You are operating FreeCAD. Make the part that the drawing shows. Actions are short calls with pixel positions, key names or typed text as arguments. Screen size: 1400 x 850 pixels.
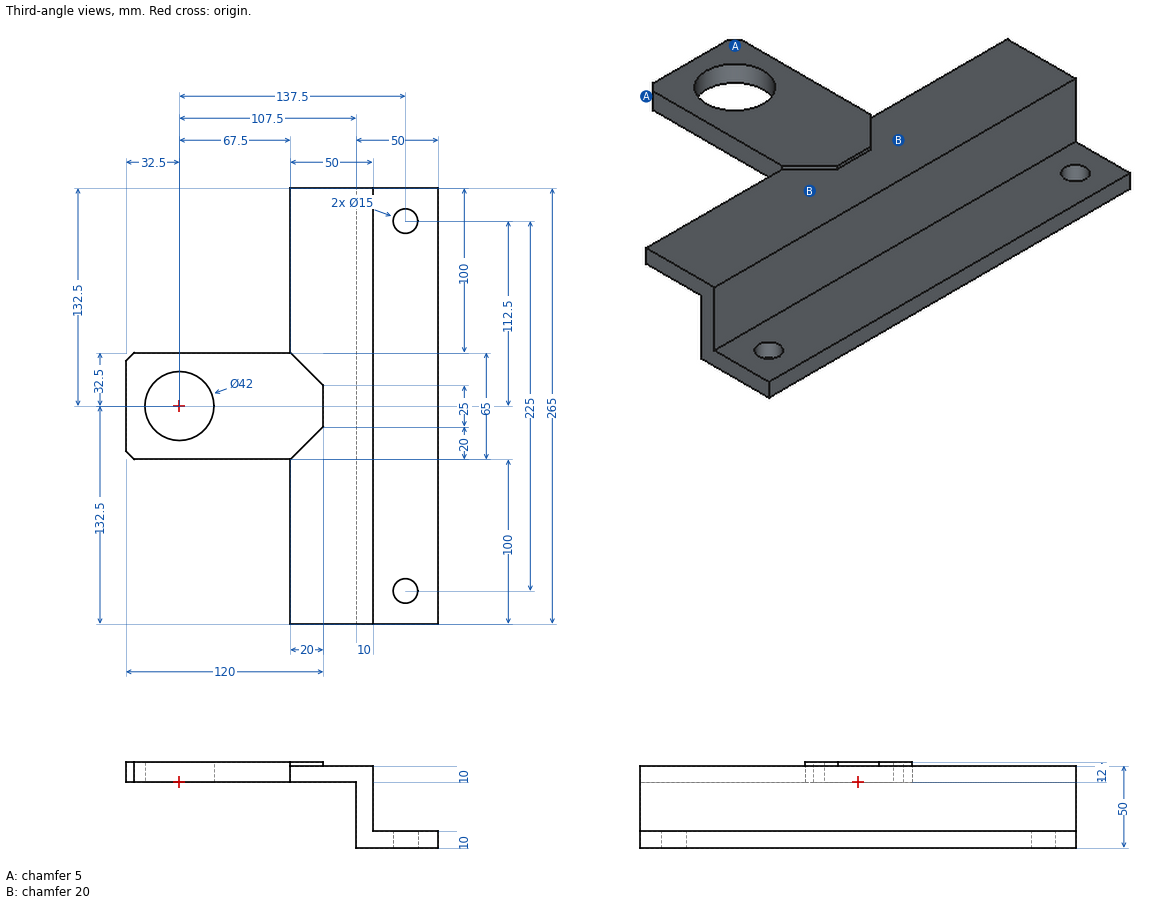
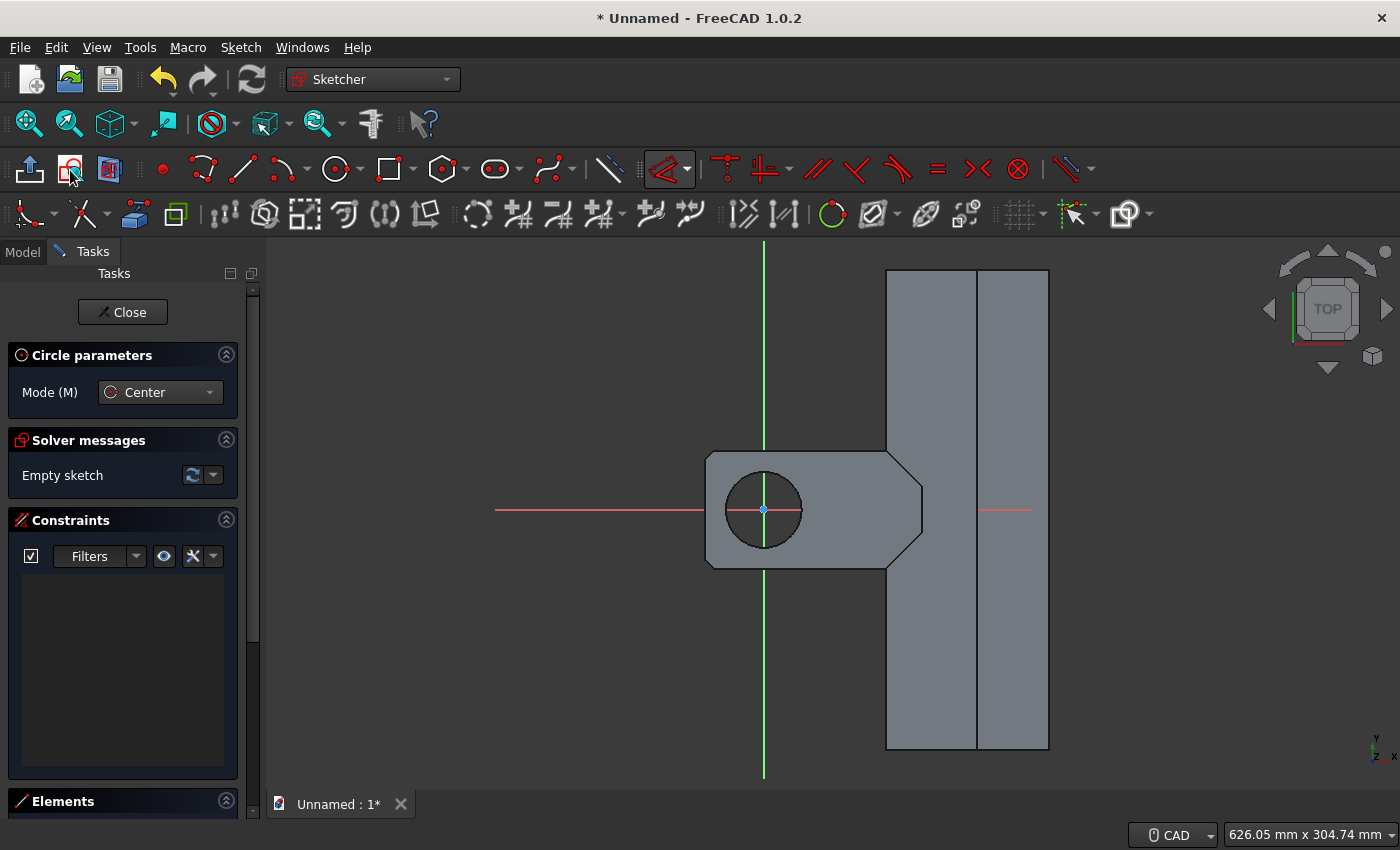
scroll(1013, 306, up, 3)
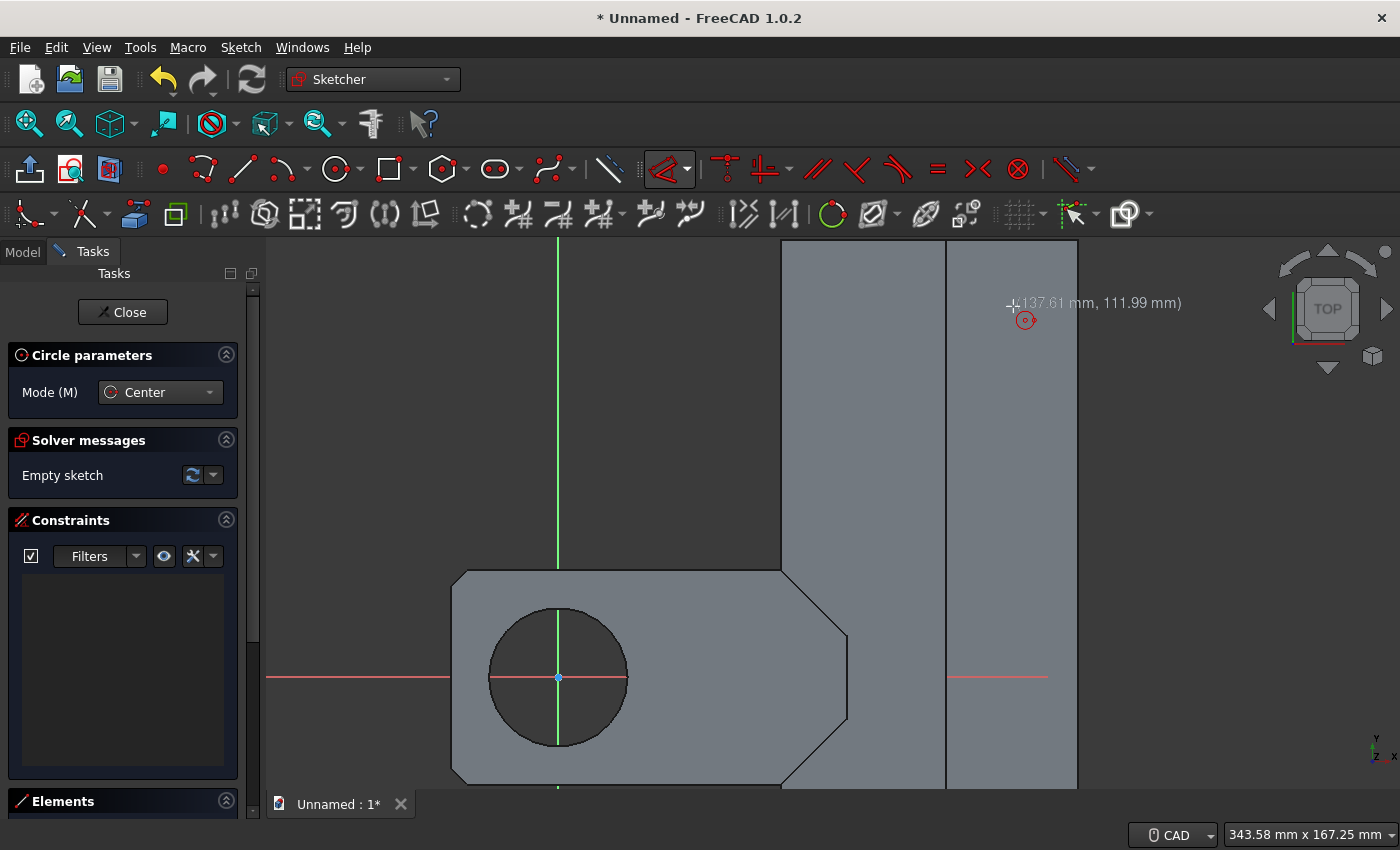
click(1012, 306)
move(1030, 289)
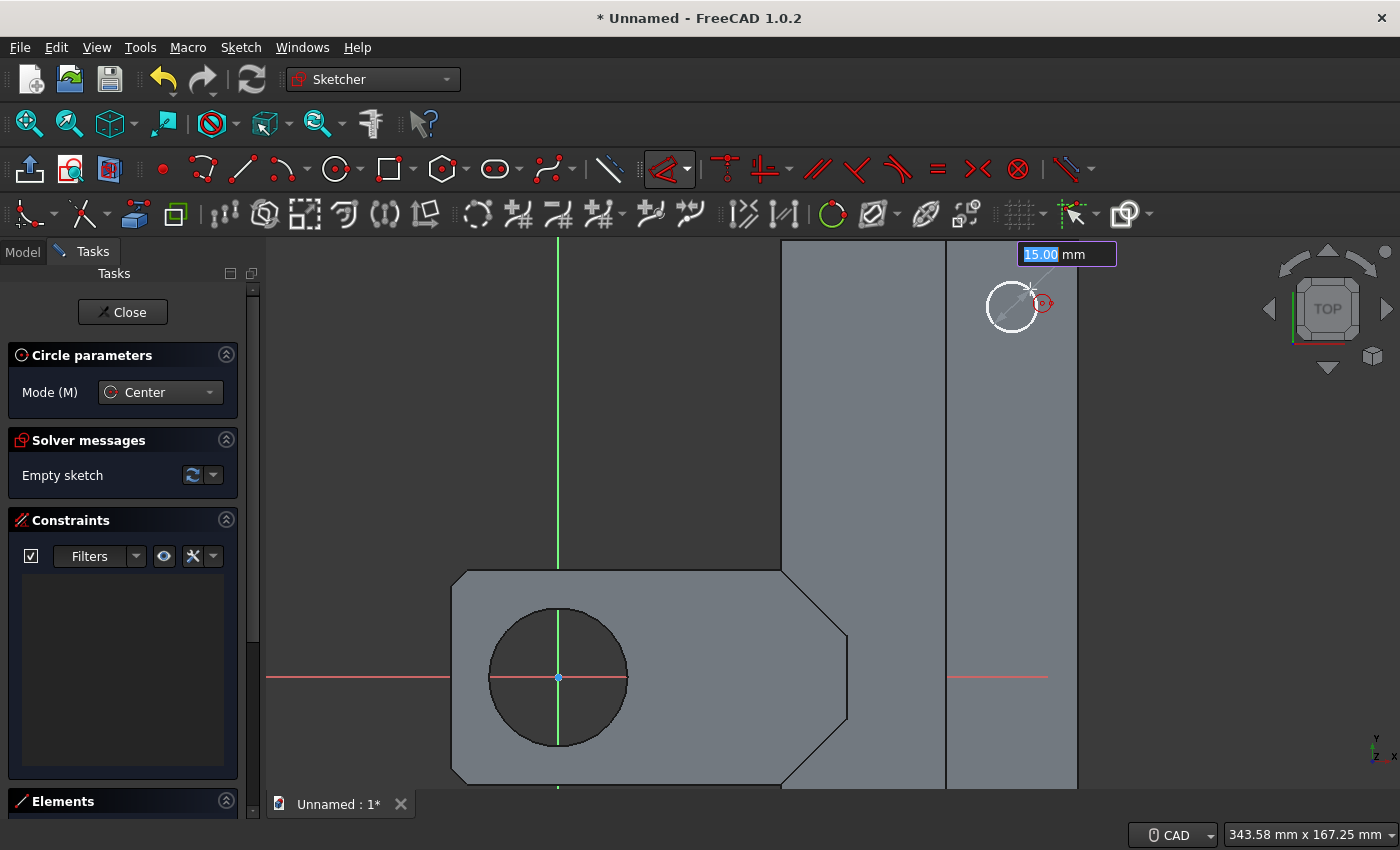
text(15)
key(Return)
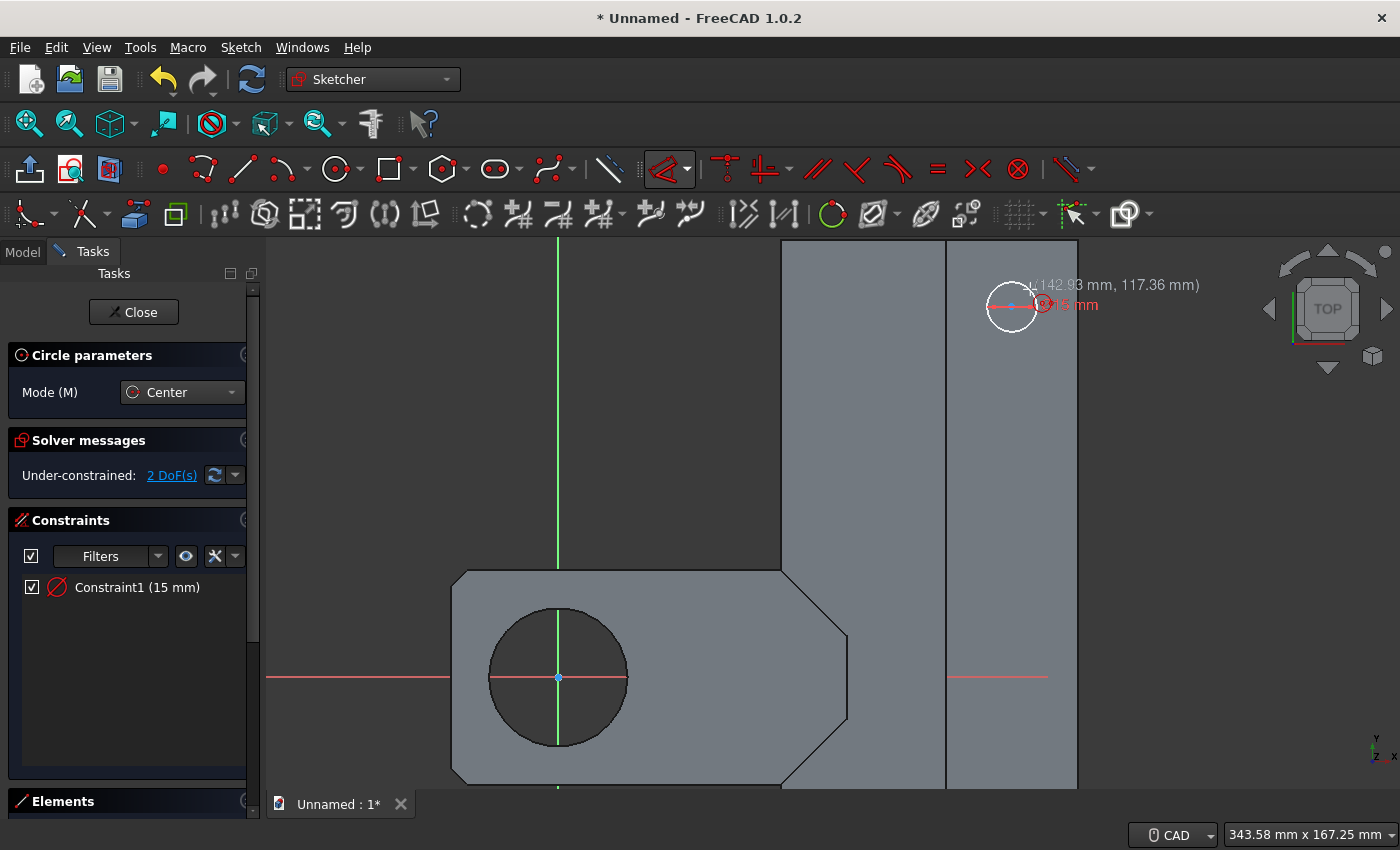
scroll(738, 379, down, 4)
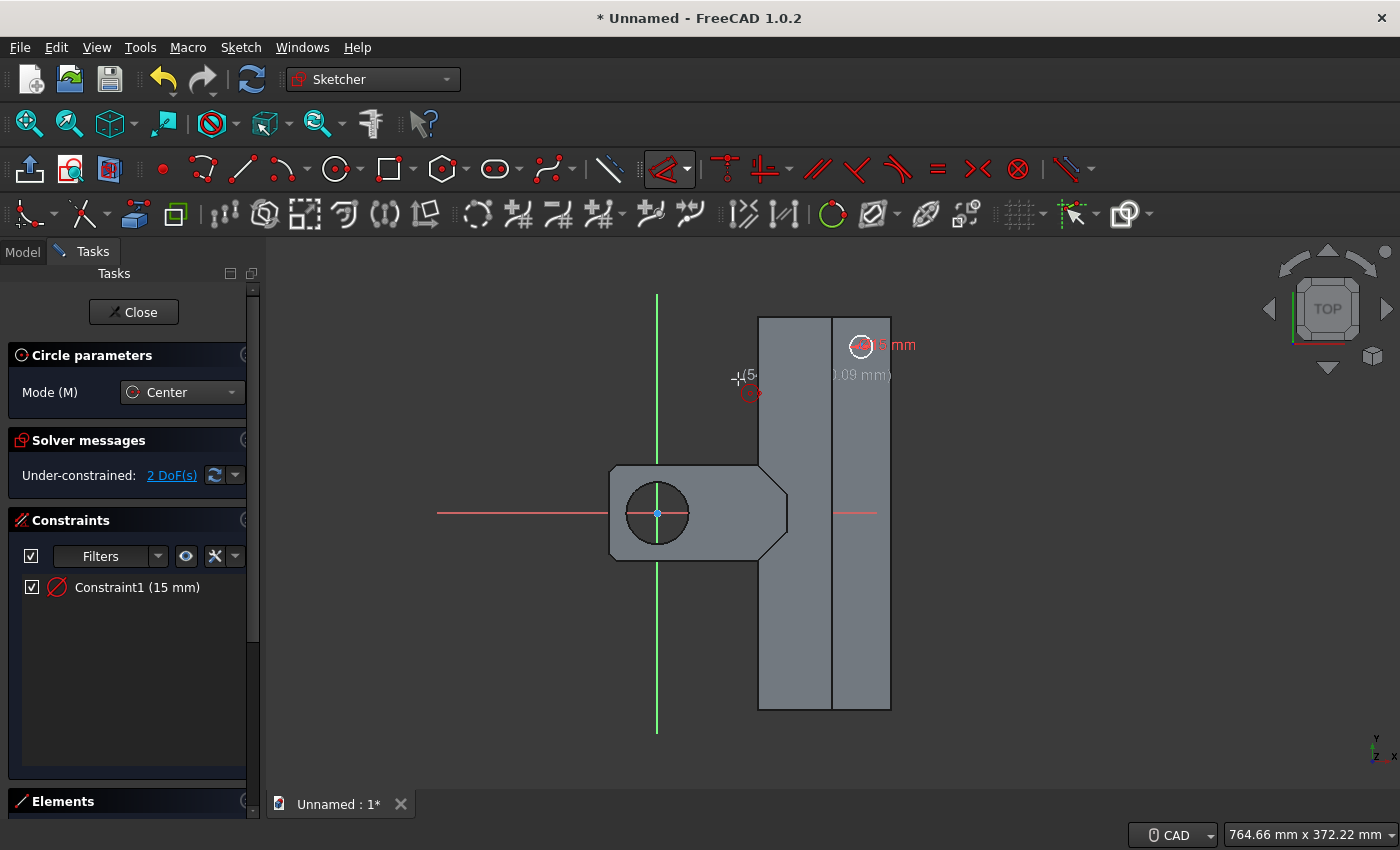
scroll(861, 680, up, 4)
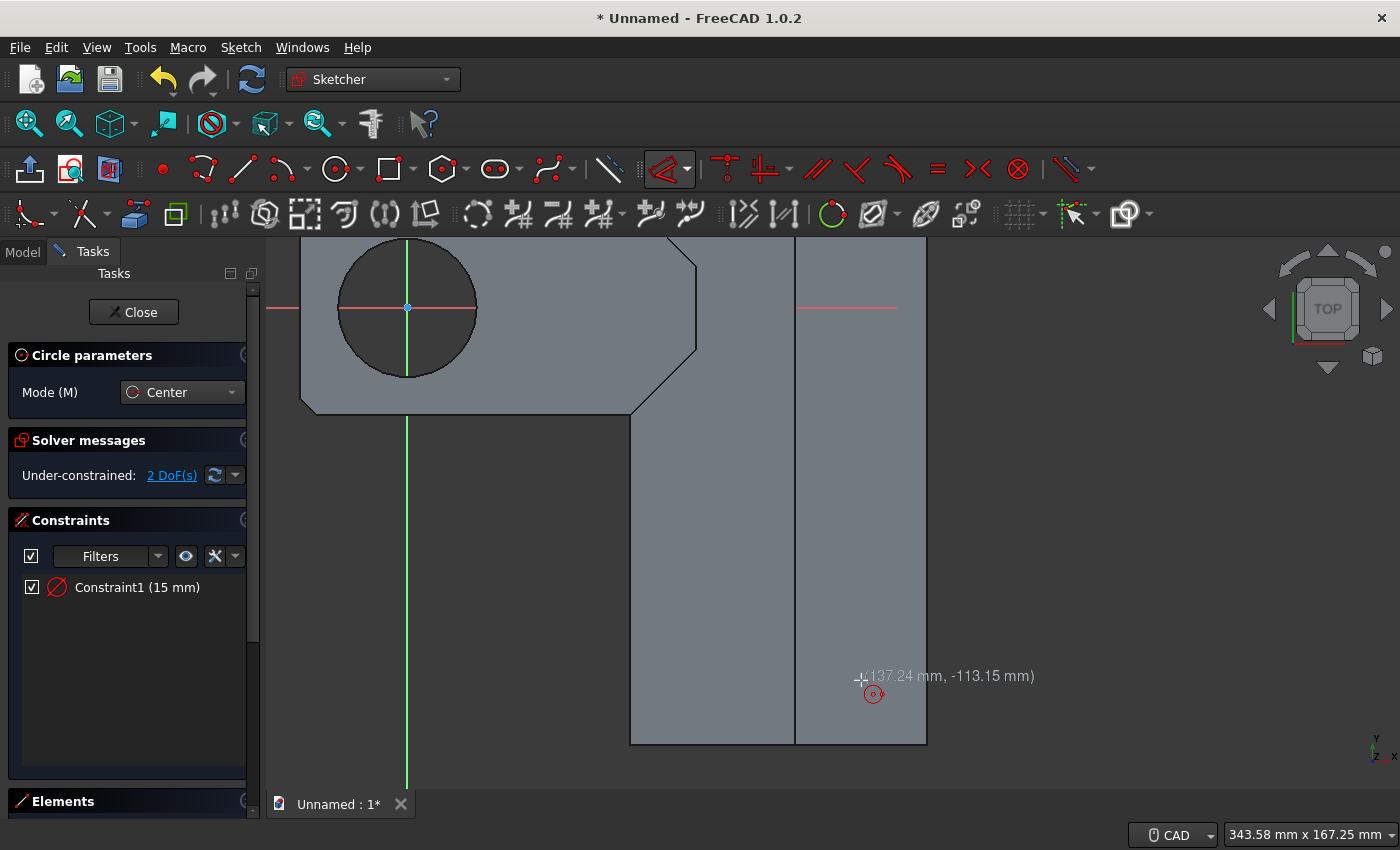
click(861, 679)
move(879, 662)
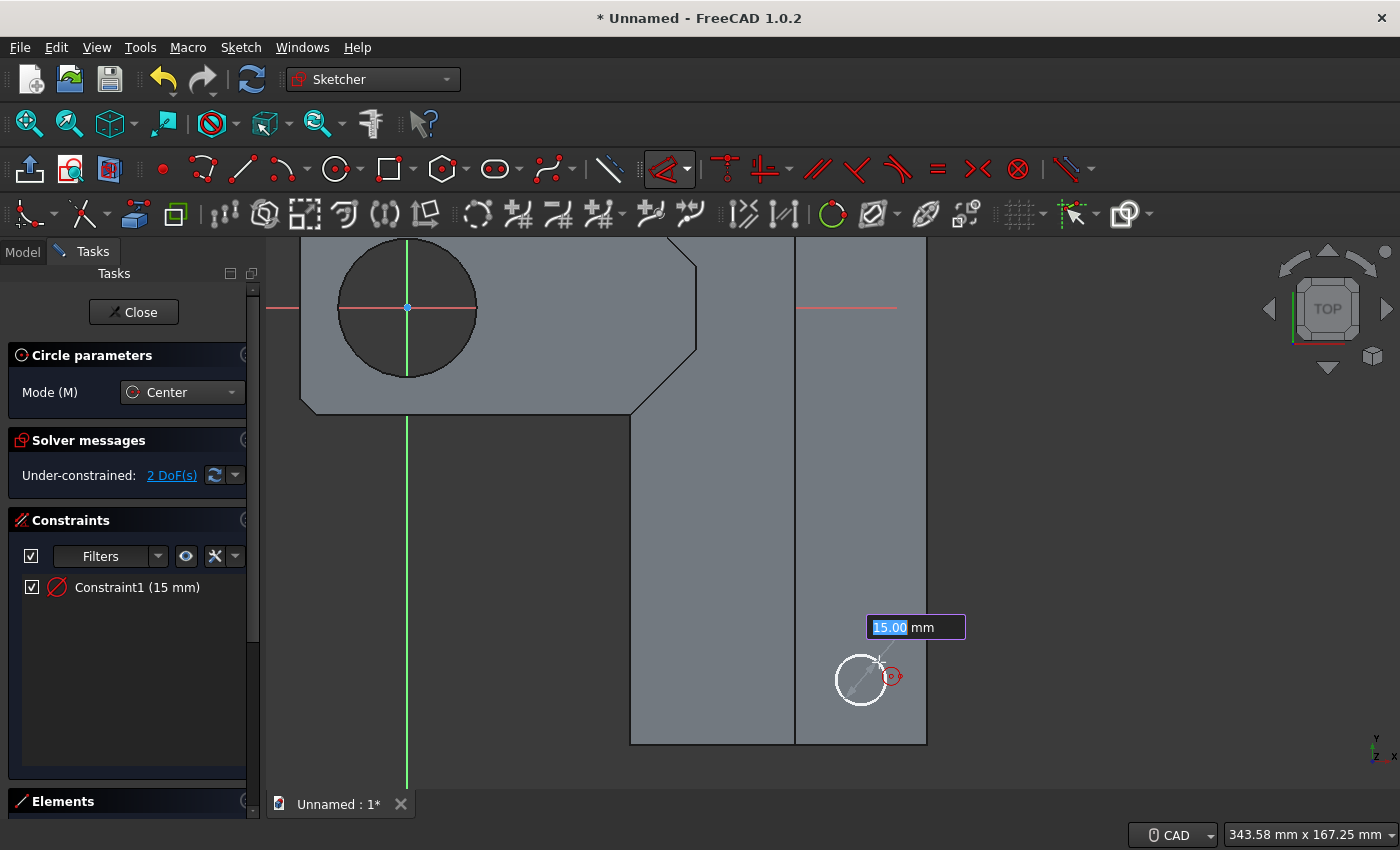
text(15)
key(Return)
key(Escape)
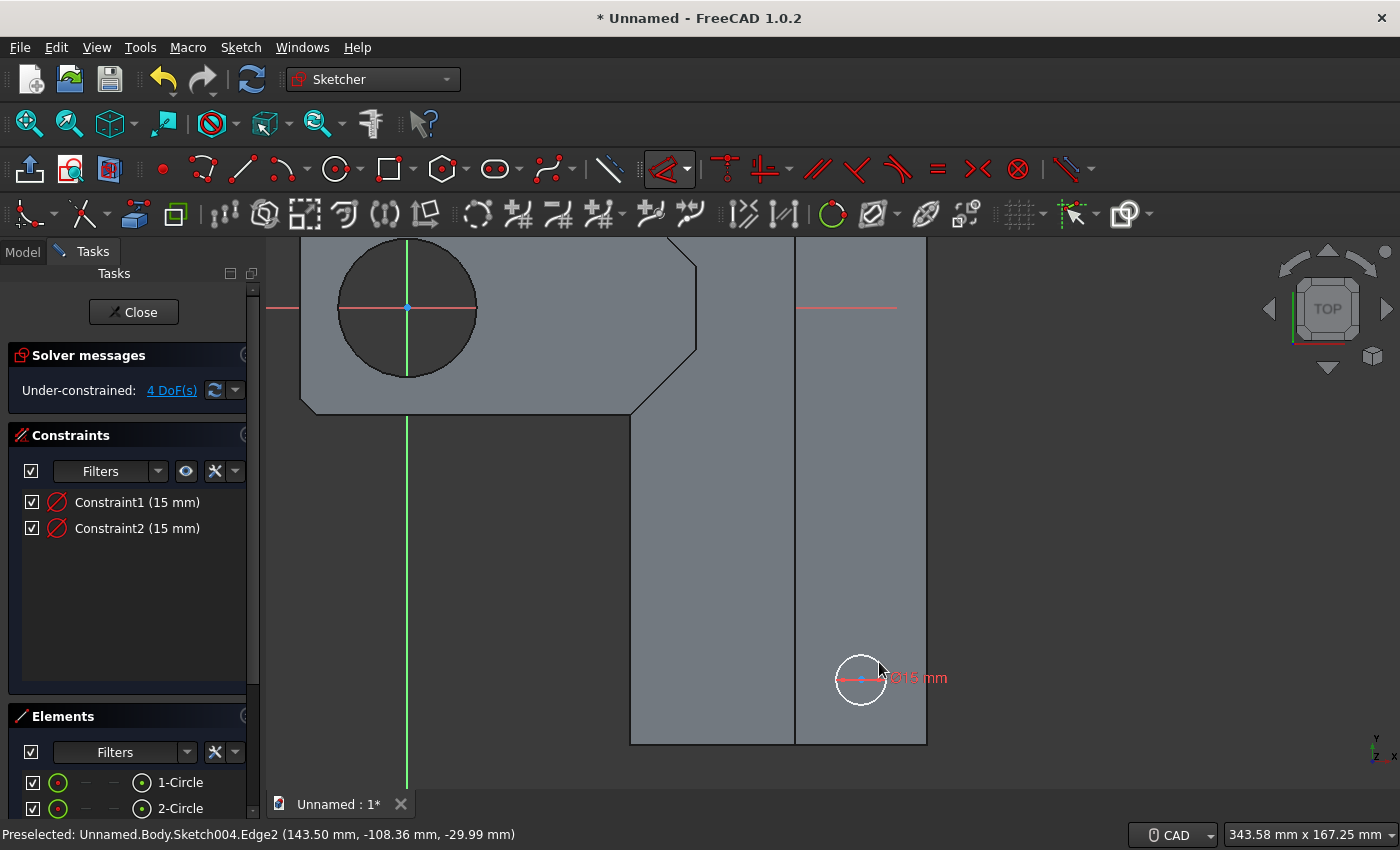
scroll(861, 680, down, 4)